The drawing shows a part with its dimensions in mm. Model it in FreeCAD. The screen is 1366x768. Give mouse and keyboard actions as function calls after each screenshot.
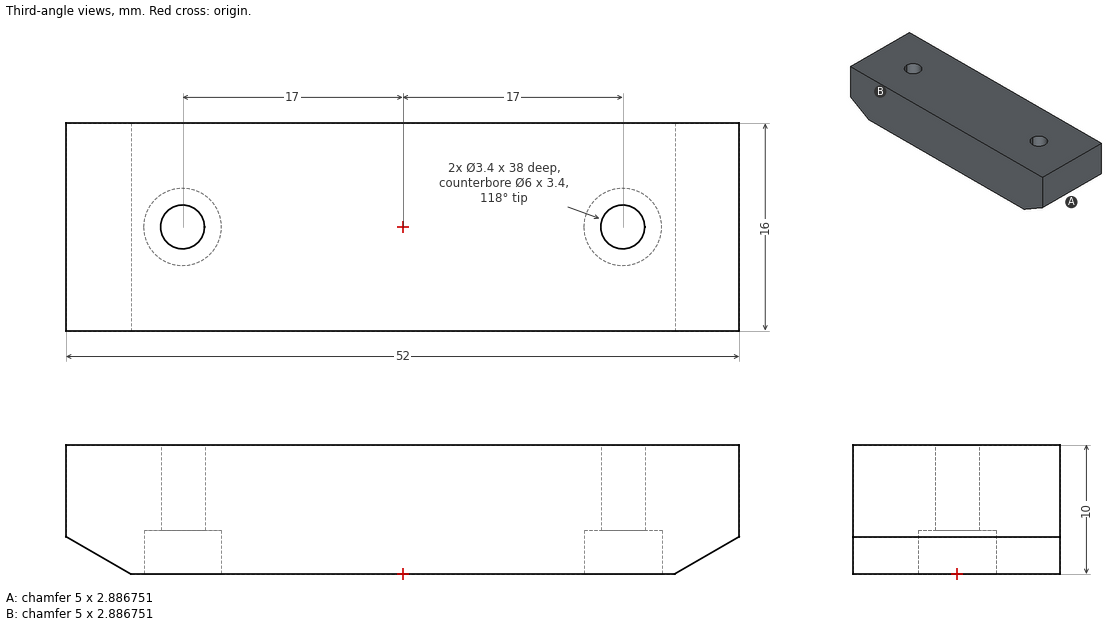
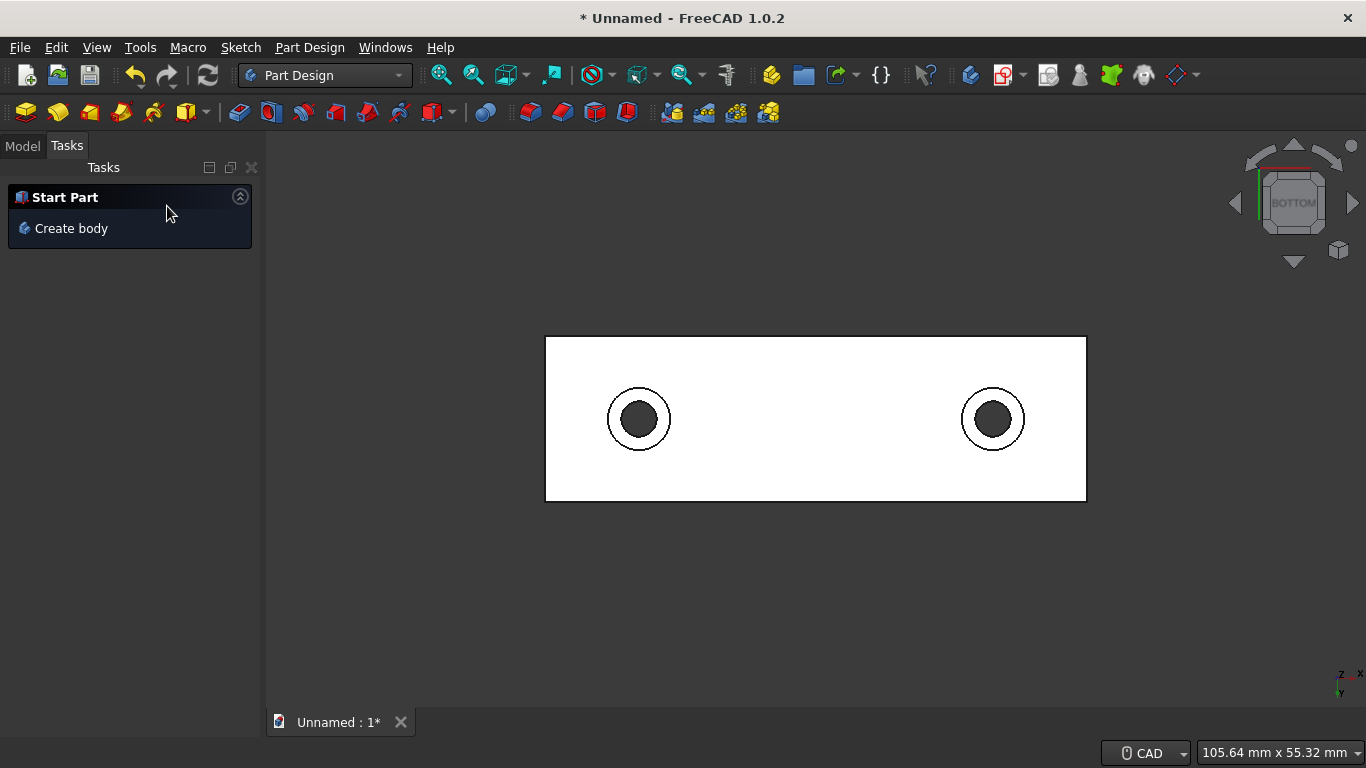
click(1087, 401)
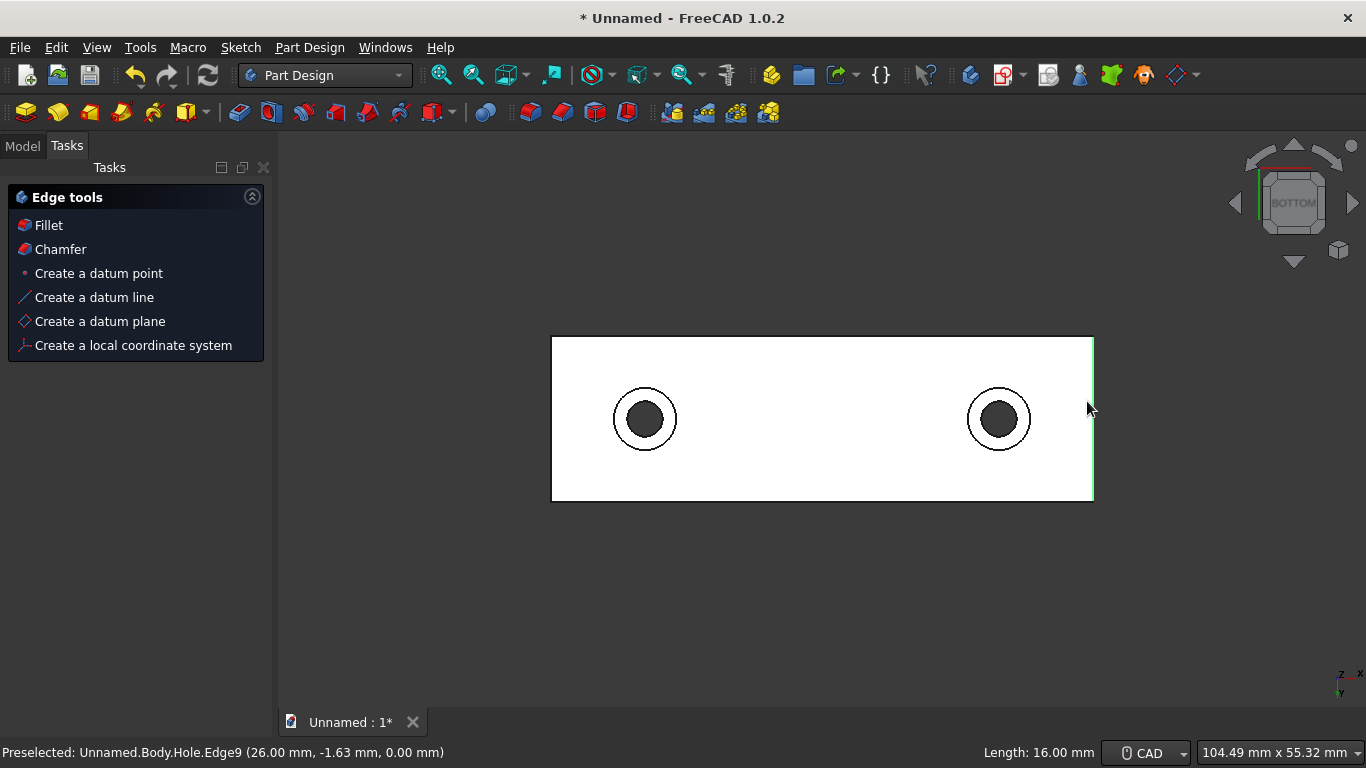
click(564, 112)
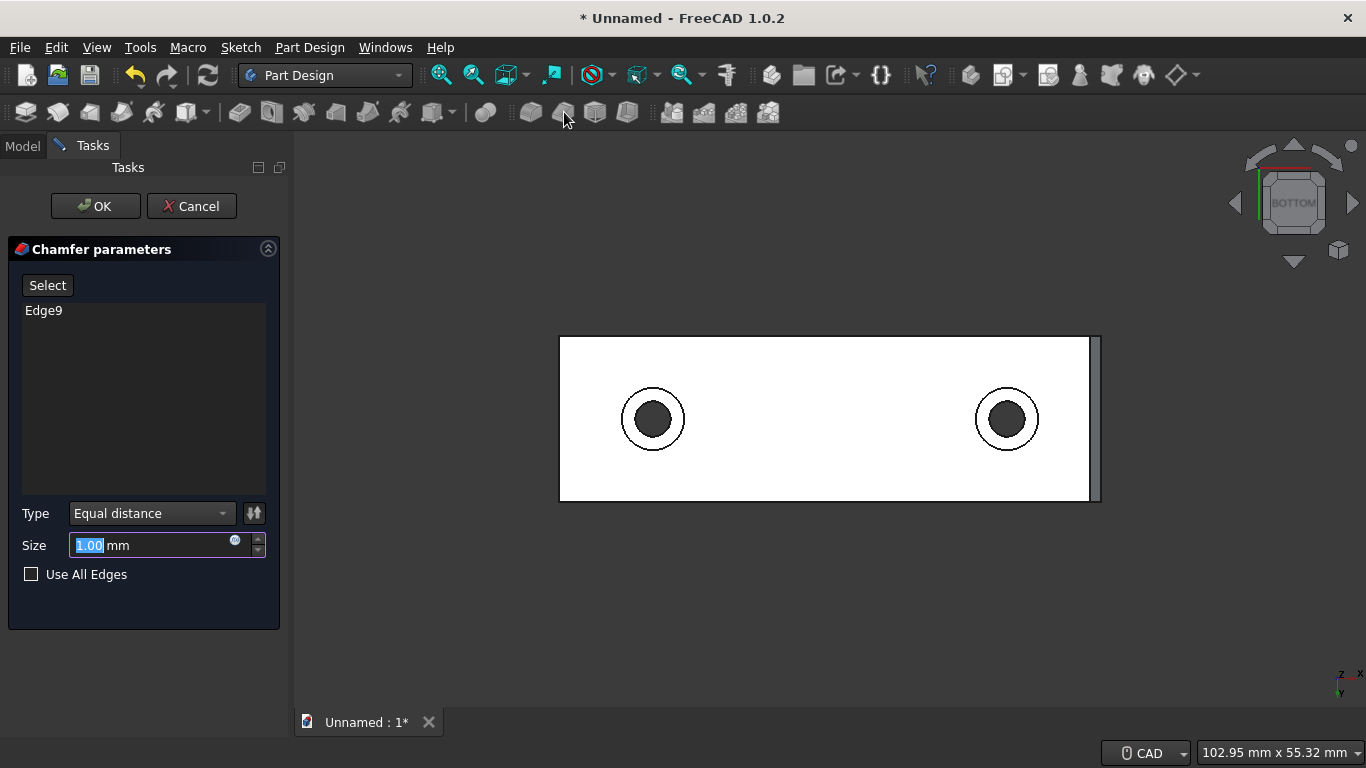
text(5)
key(Tab)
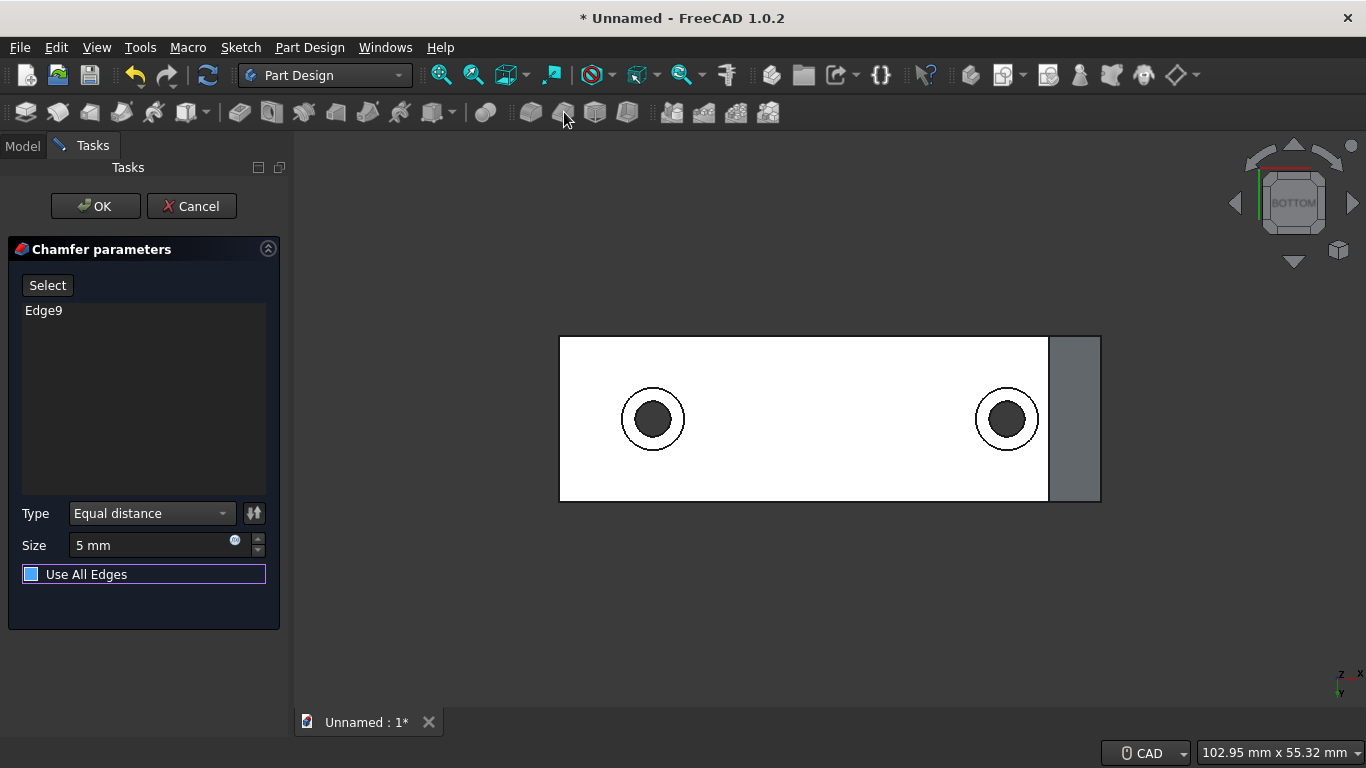
click(153, 514)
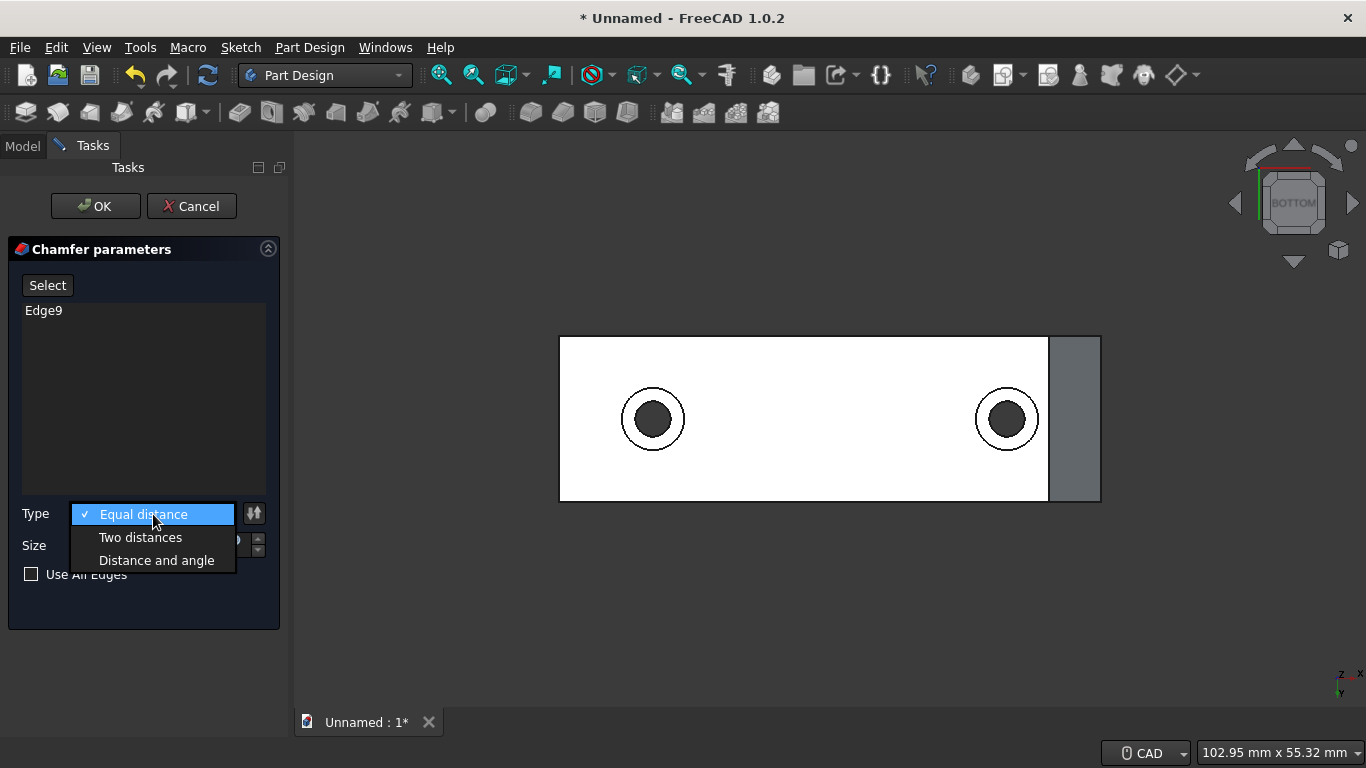
click(152, 538)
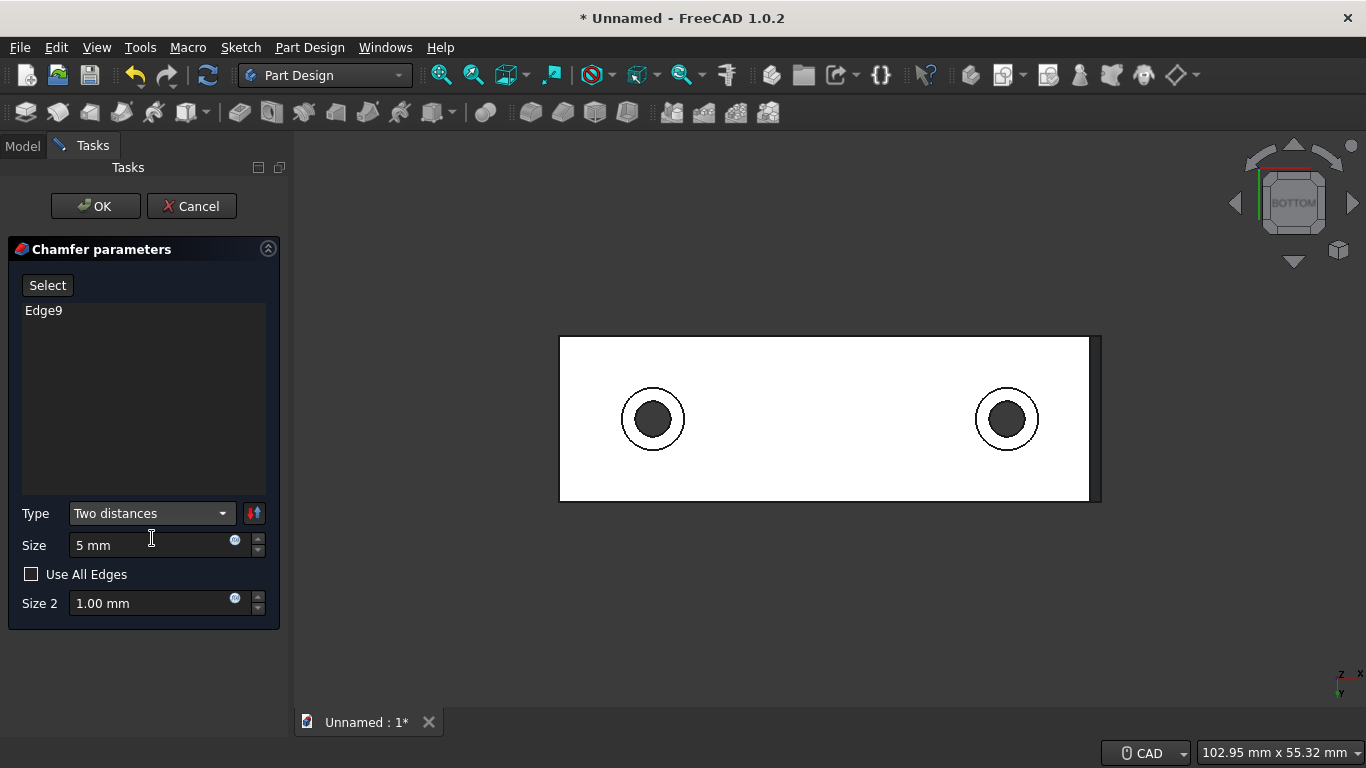
triple_click(160, 603)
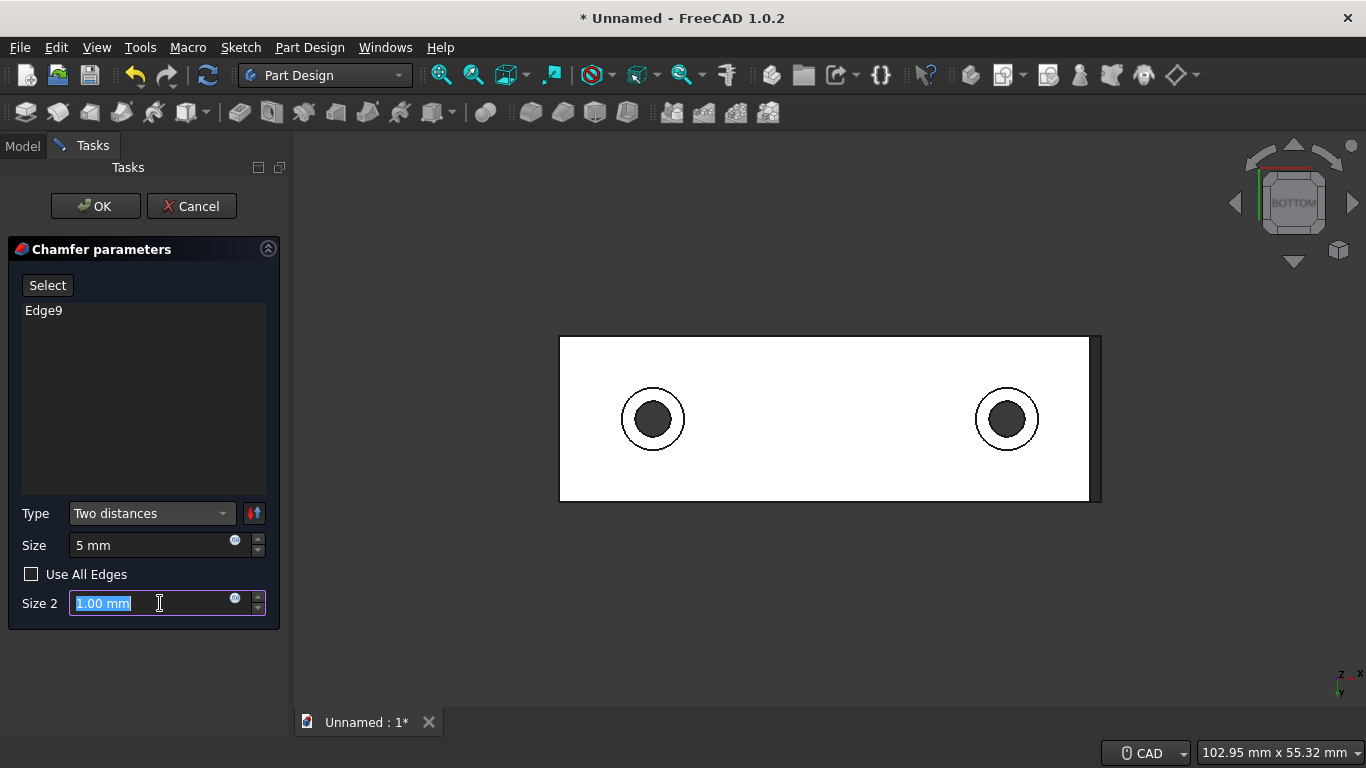
text(2.886751)
key(Tab)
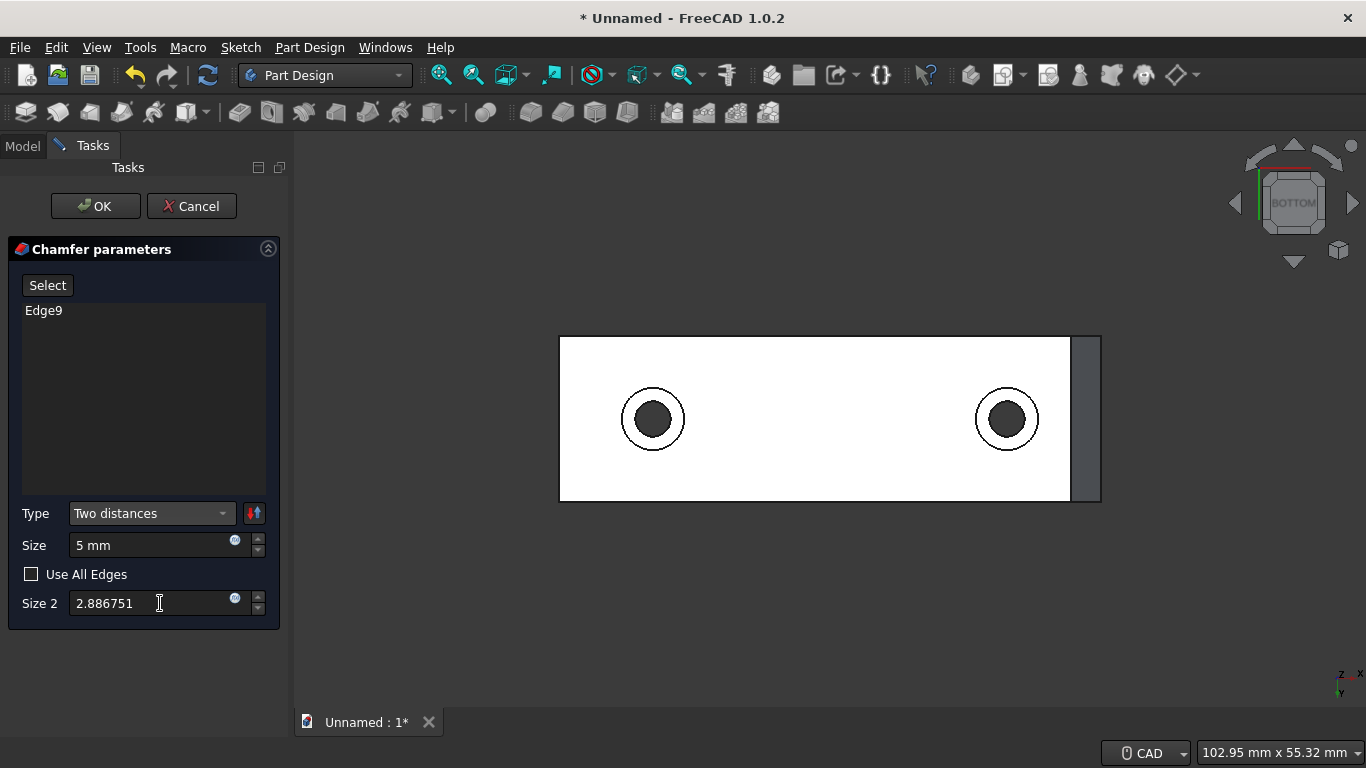
click(254, 514)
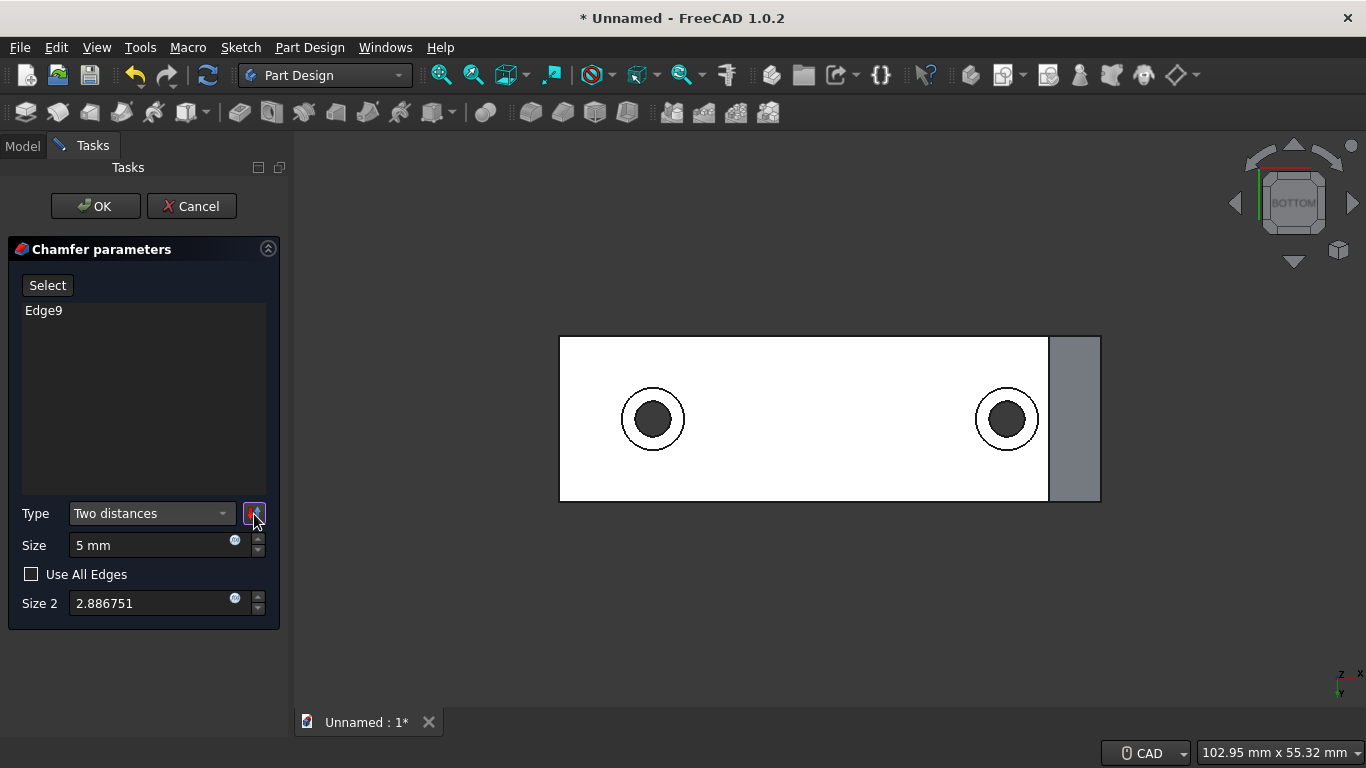
click(96, 206)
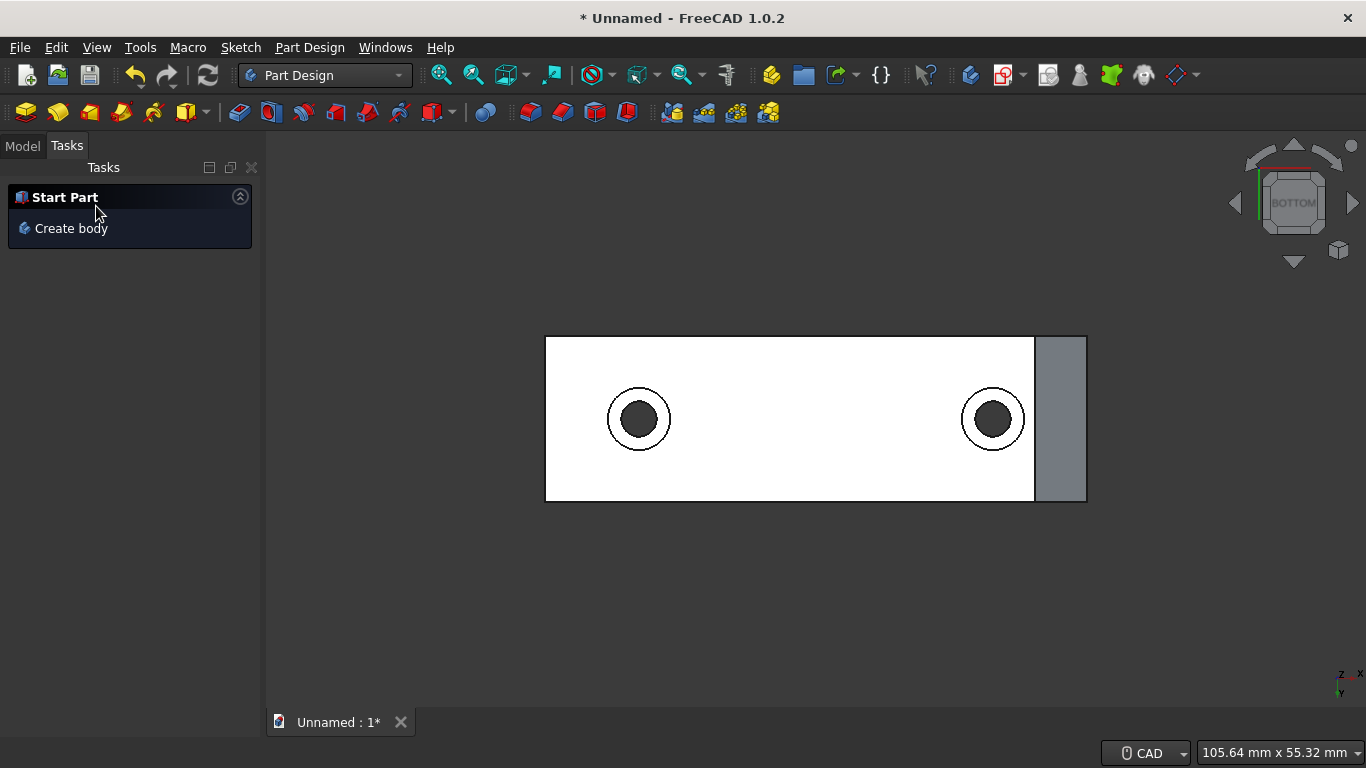
click(545, 418)